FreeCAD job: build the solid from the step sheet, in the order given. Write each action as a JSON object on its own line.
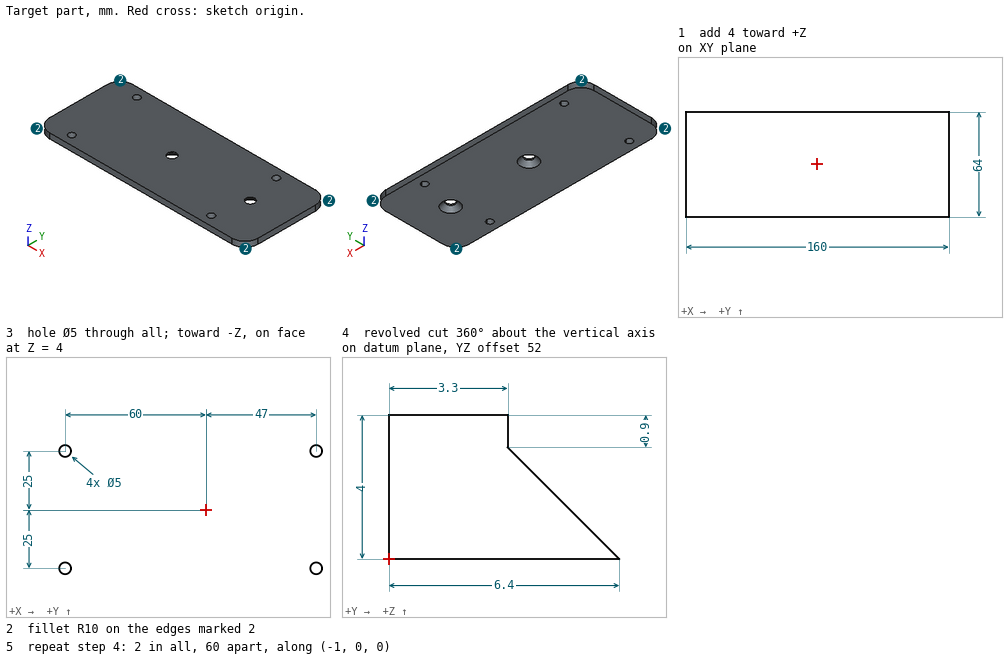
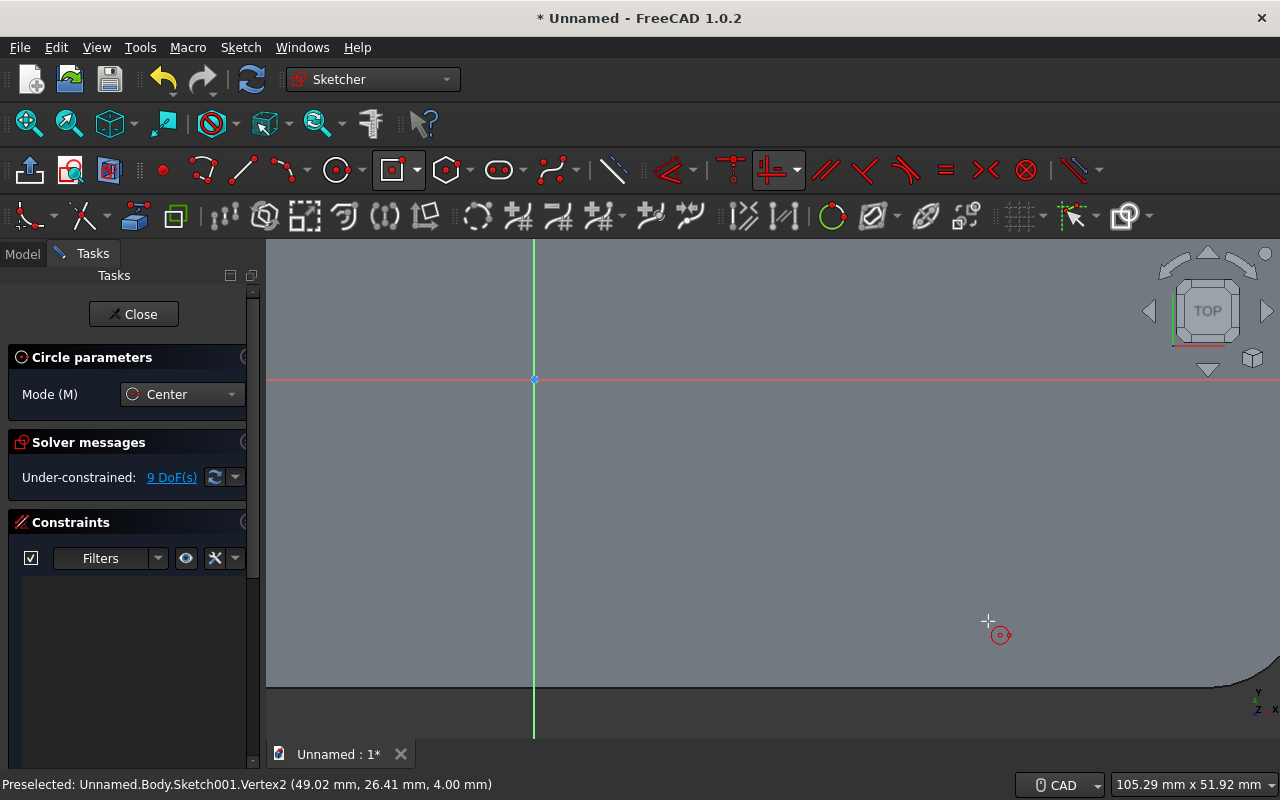
{"action": "left_click", "coordinate": [987, 621]}
{"action": "left_click", "coordinate": [1004, 604]}
{"action": "key", "text": "Escape"}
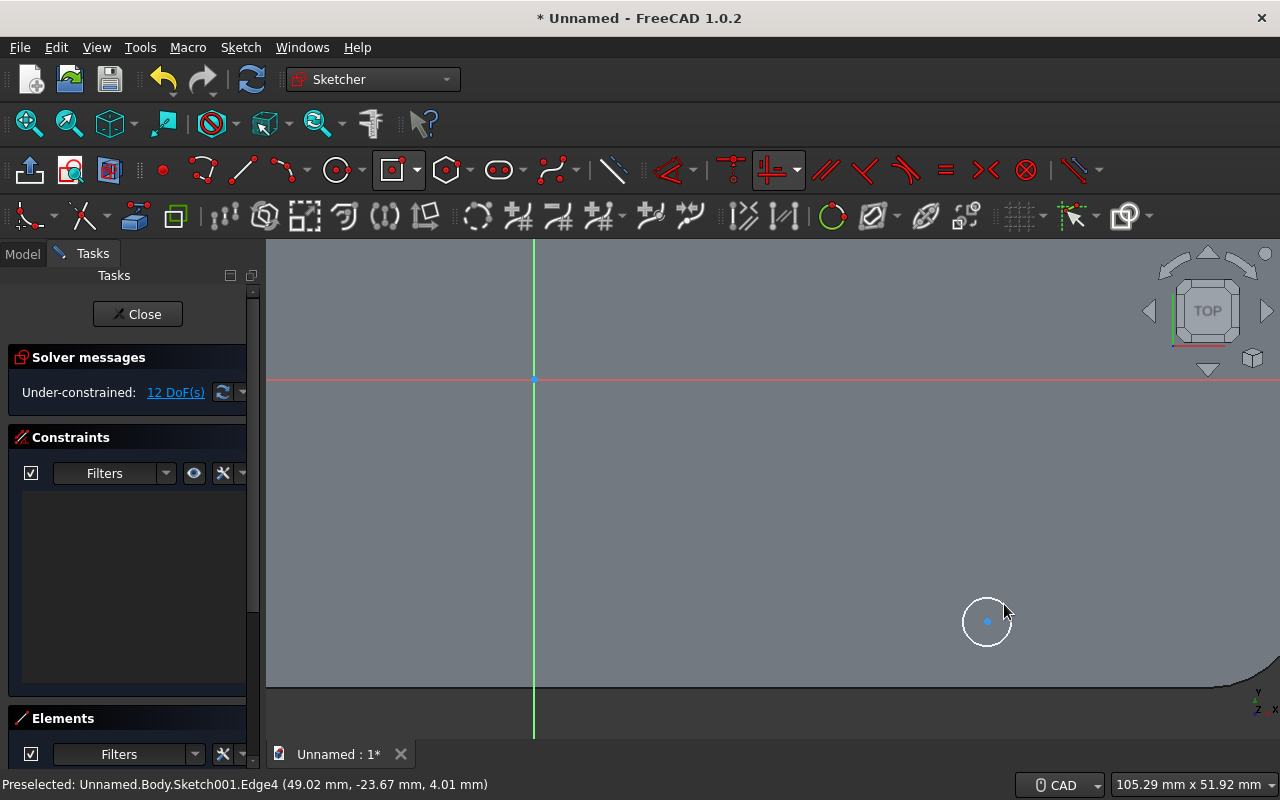
{"action": "scroll", "coordinate": [988, 622], "scroll_direction": "down", "scroll_amount": 3}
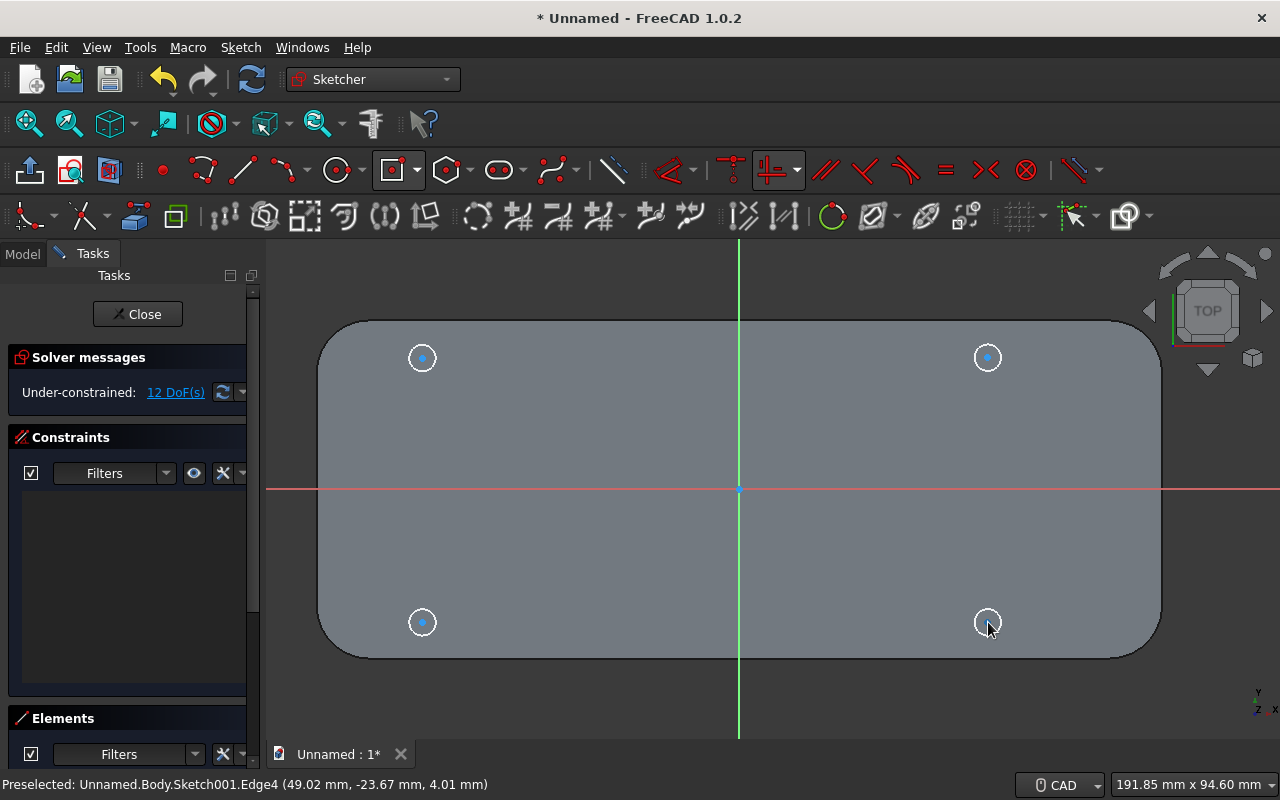
{"action": "left_click", "coordinate": [432, 349]}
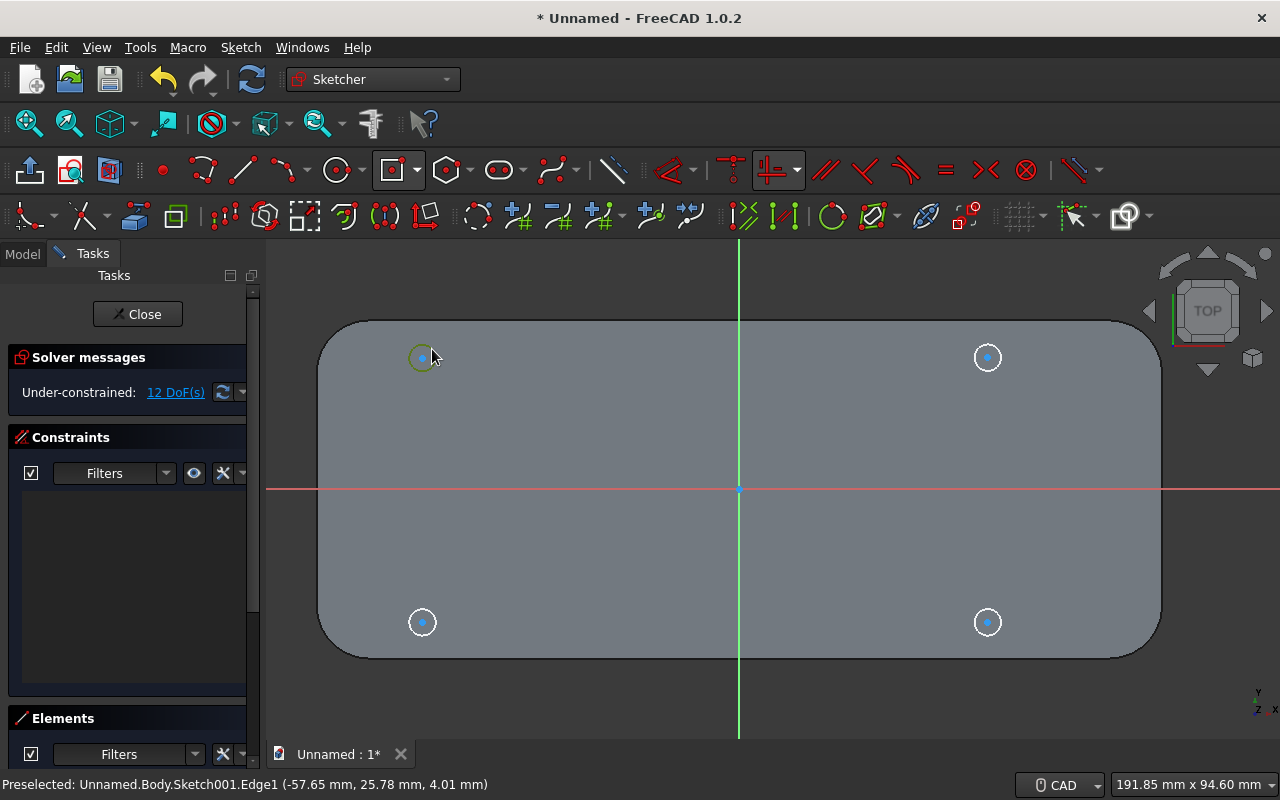
{"action": "left_click", "coordinate": [432, 613]}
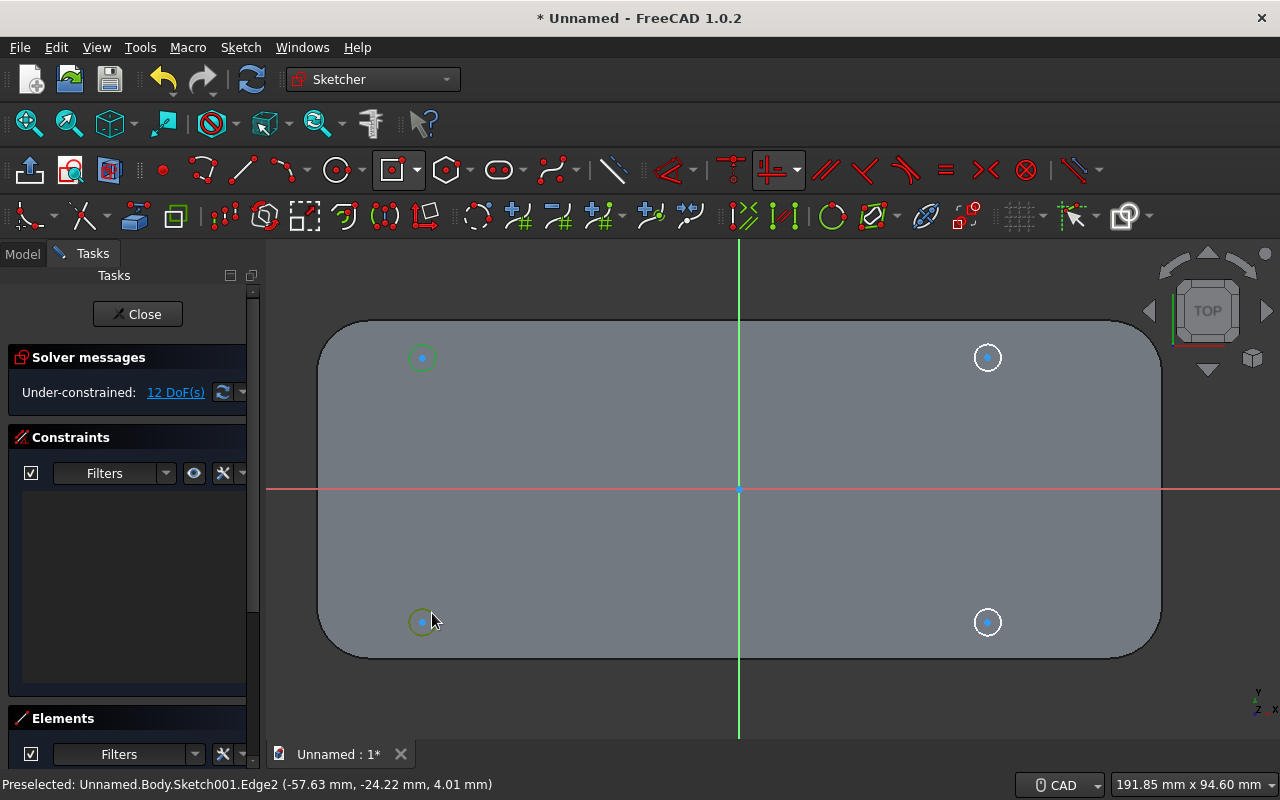
{"action": "left_click", "coordinate": [997, 348]}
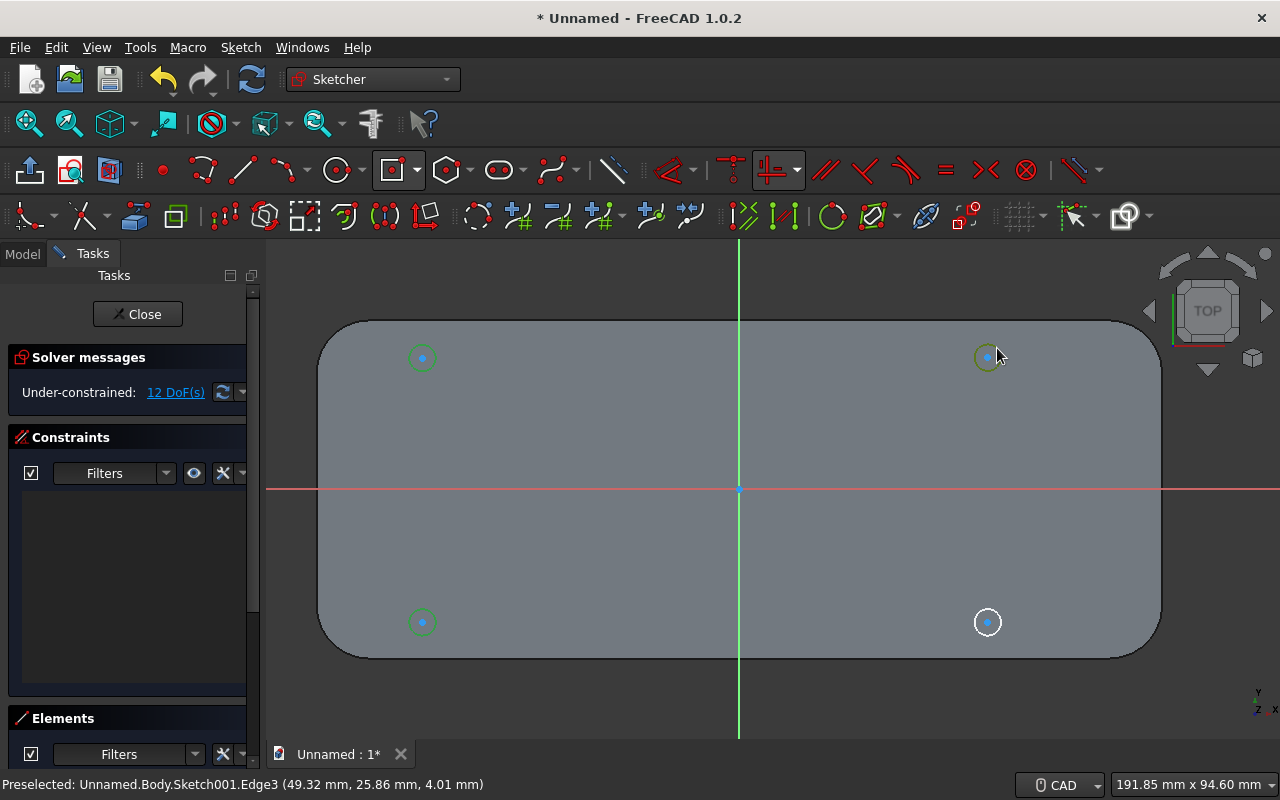
{"action": "left_click", "coordinate": [997, 613]}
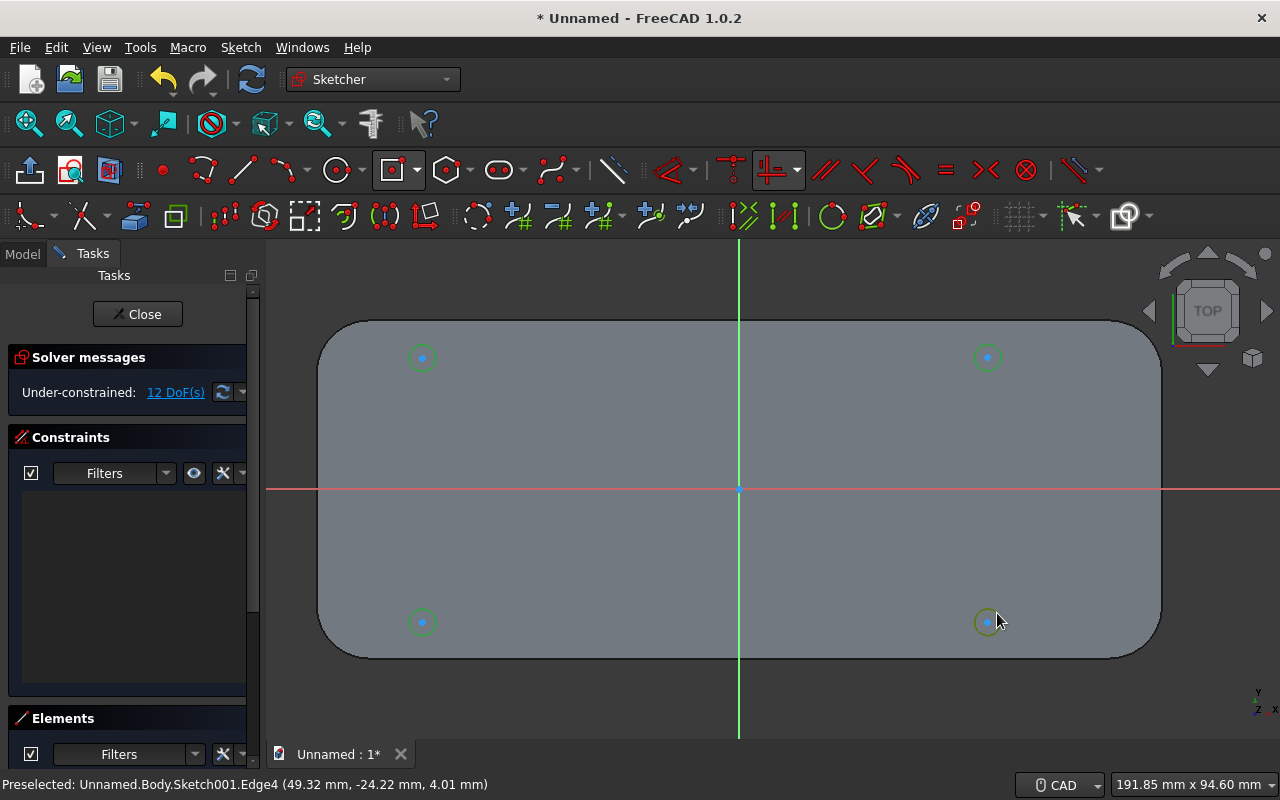
{"action": "left_click", "coordinate": [946, 170]}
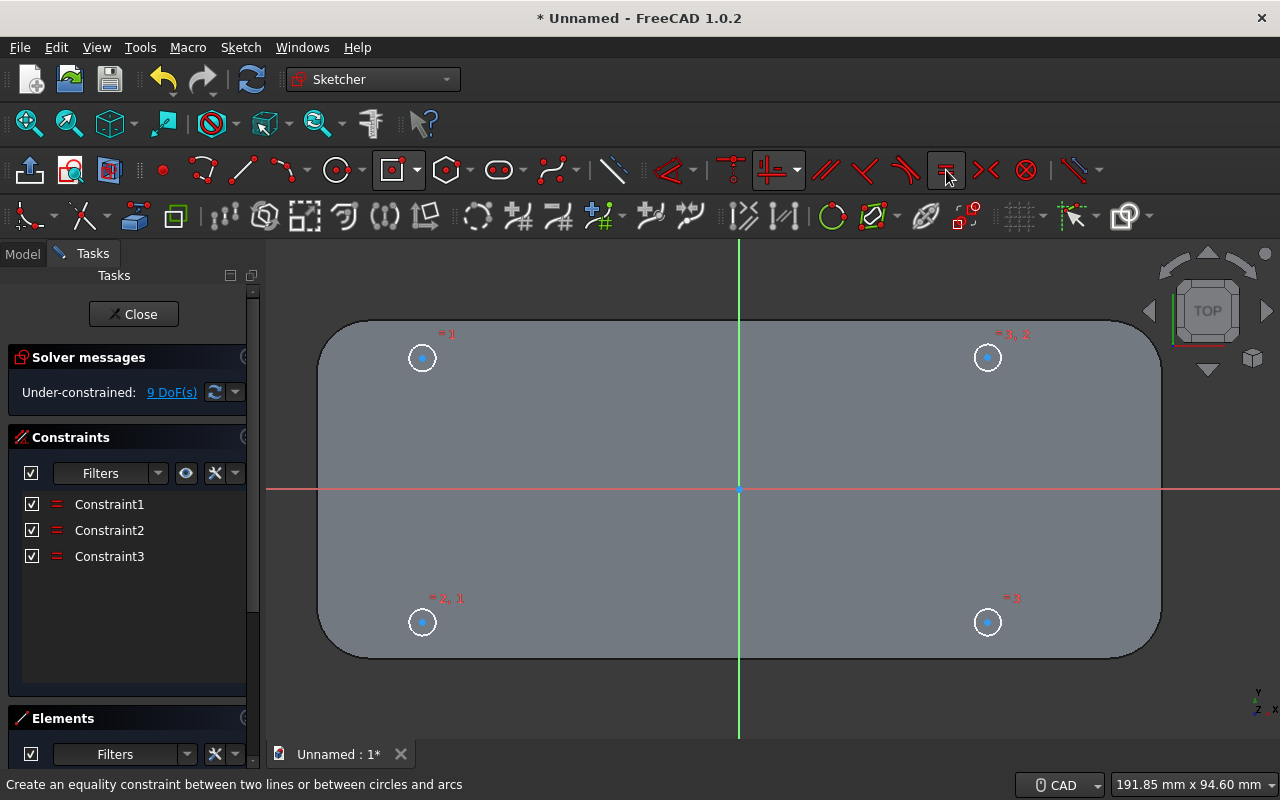
{"action": "left_click", "coordinate": [422, 358]}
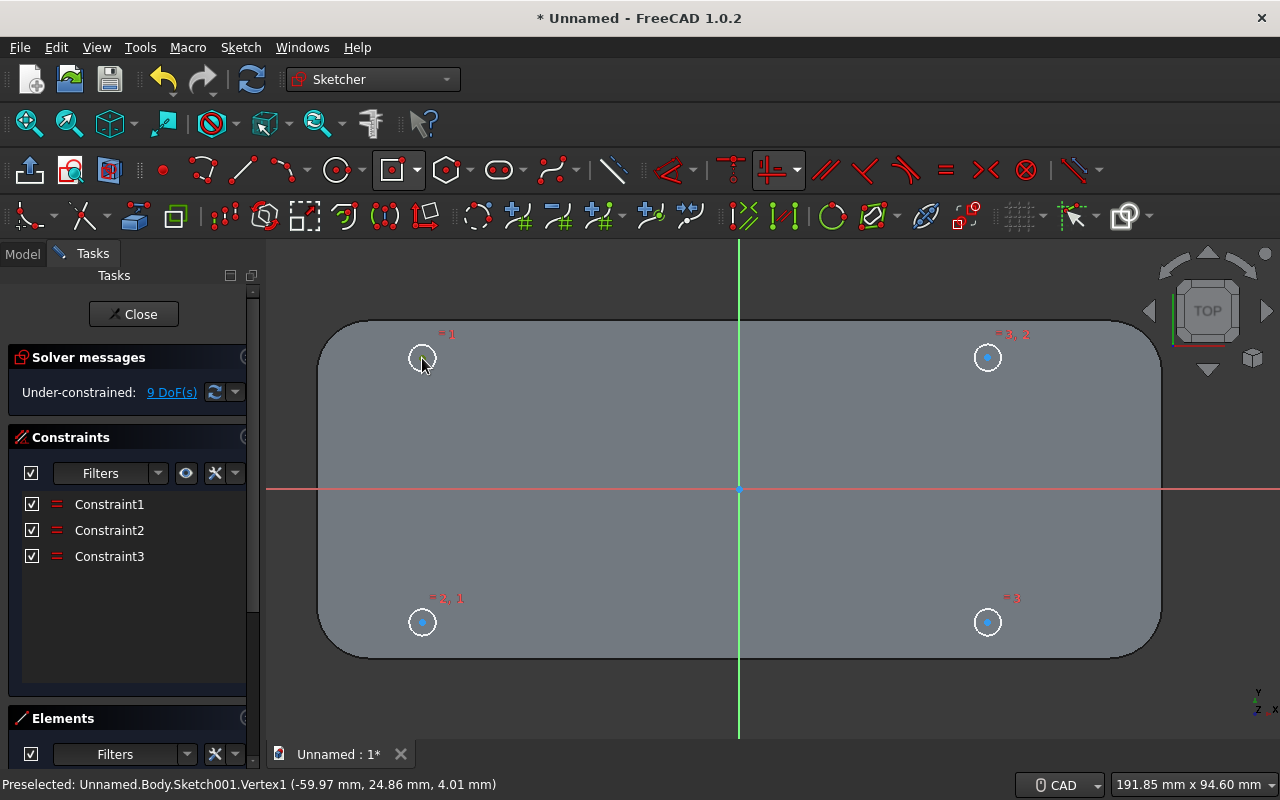
{"action": "left_click", "coordinate": [423, 622]}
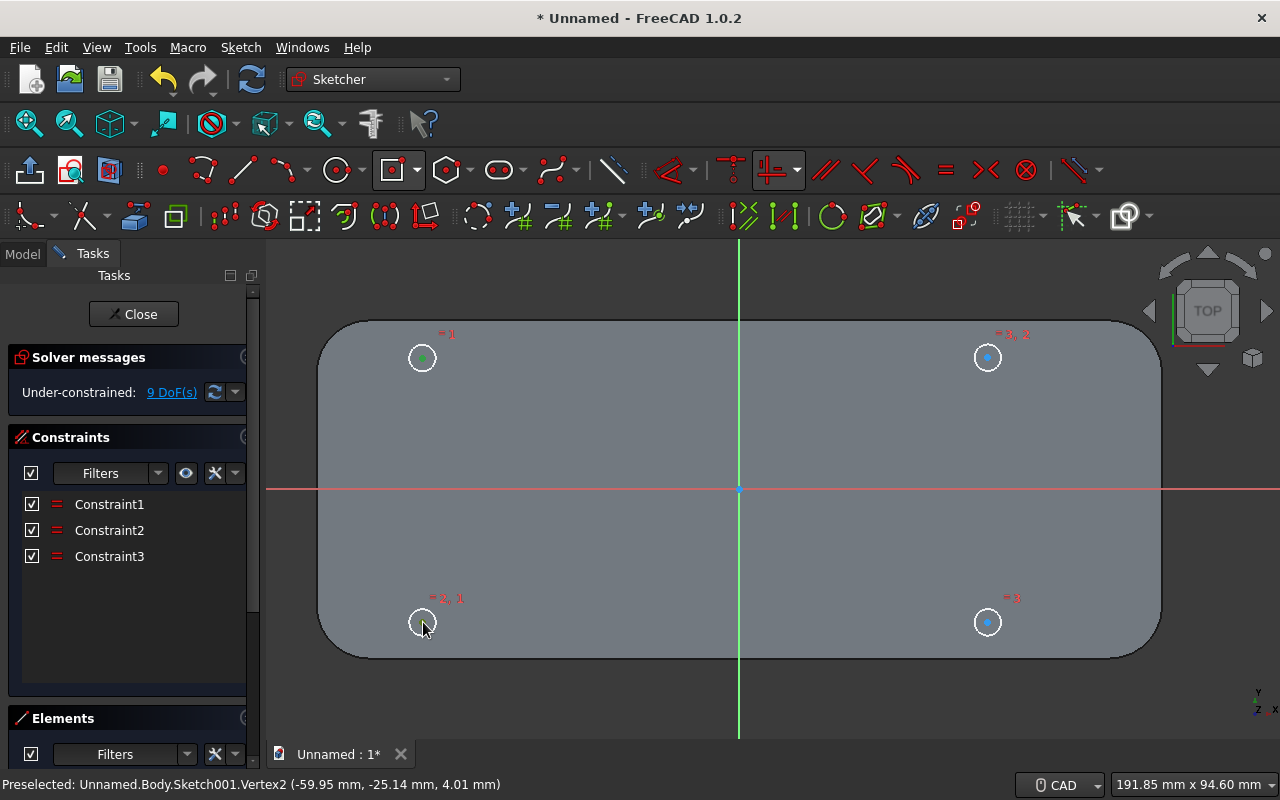
{"action": "left_click", "coordinate": [800, 170]}